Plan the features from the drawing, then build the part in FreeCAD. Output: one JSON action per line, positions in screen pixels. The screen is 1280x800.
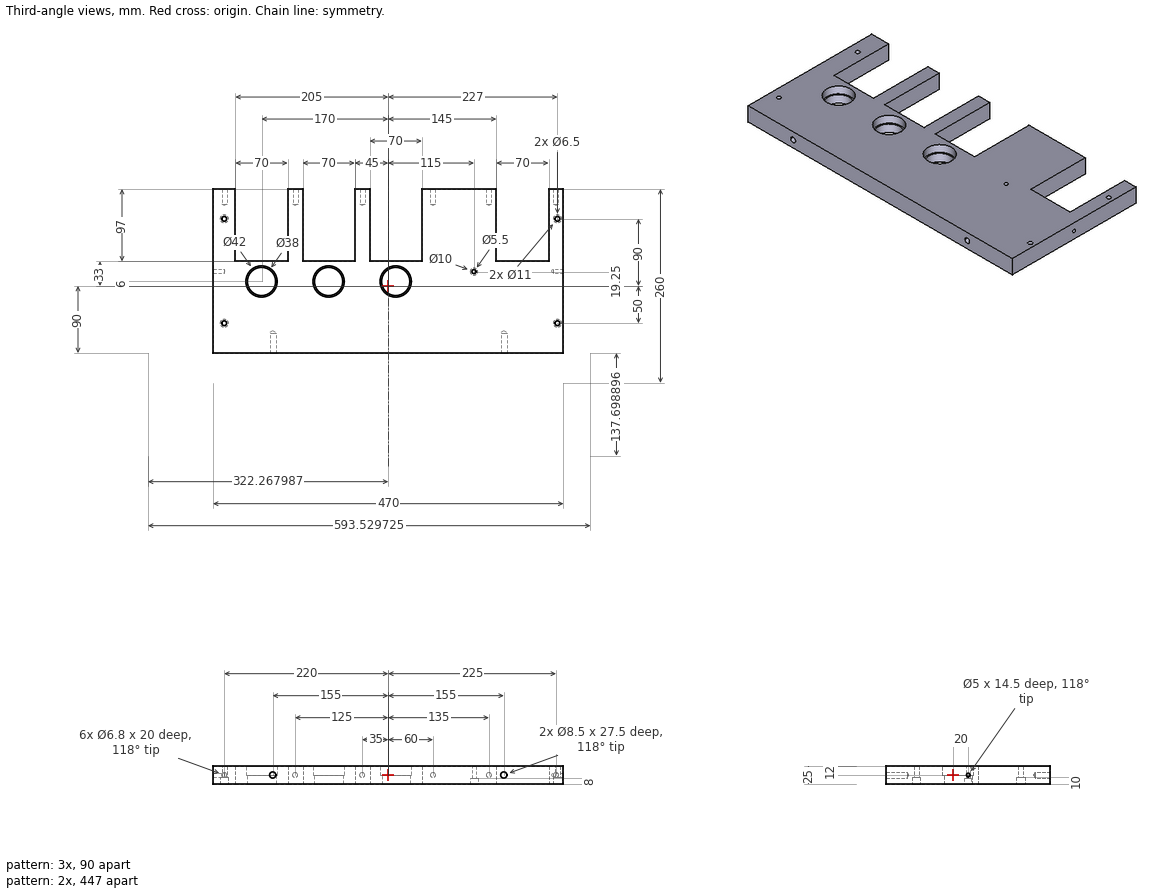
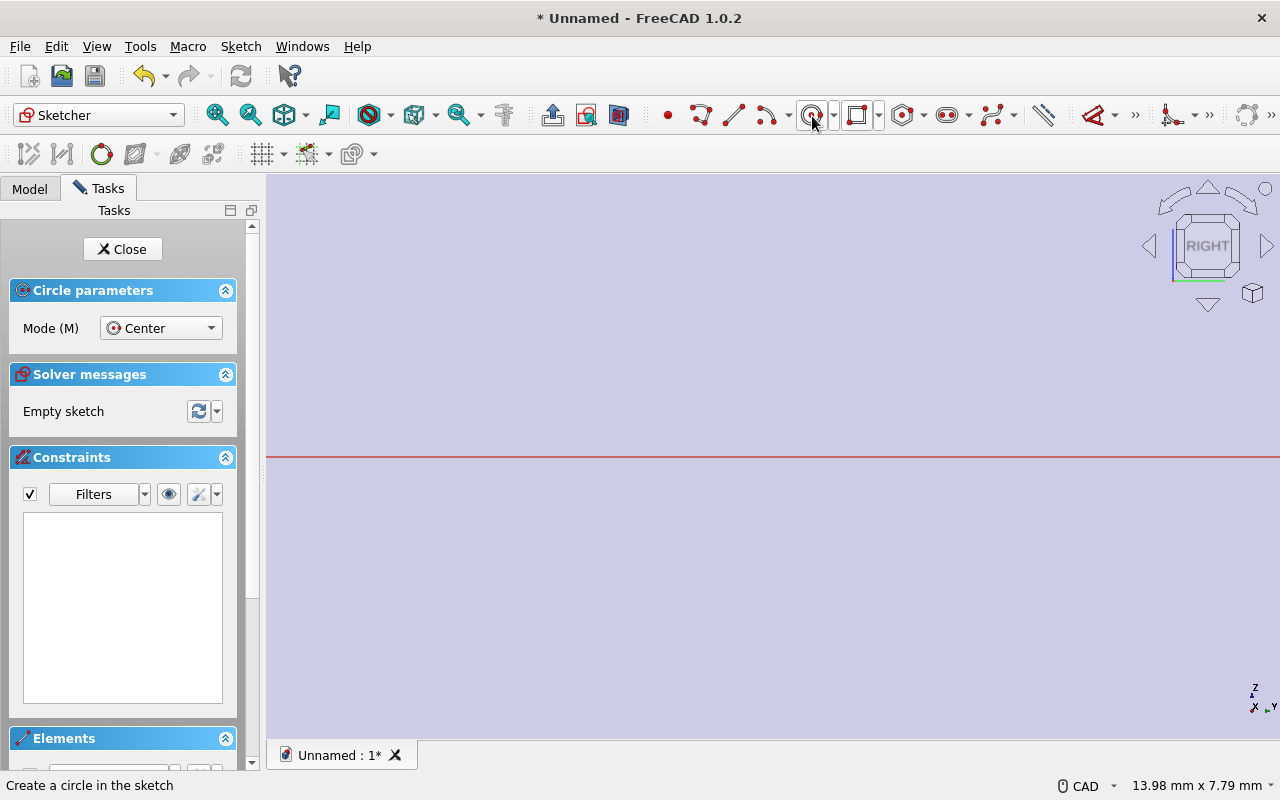
{"action": "left_click", "coordinate": [705, 456]}
{"action": "mouse_move", "coordinate": [833, 328]}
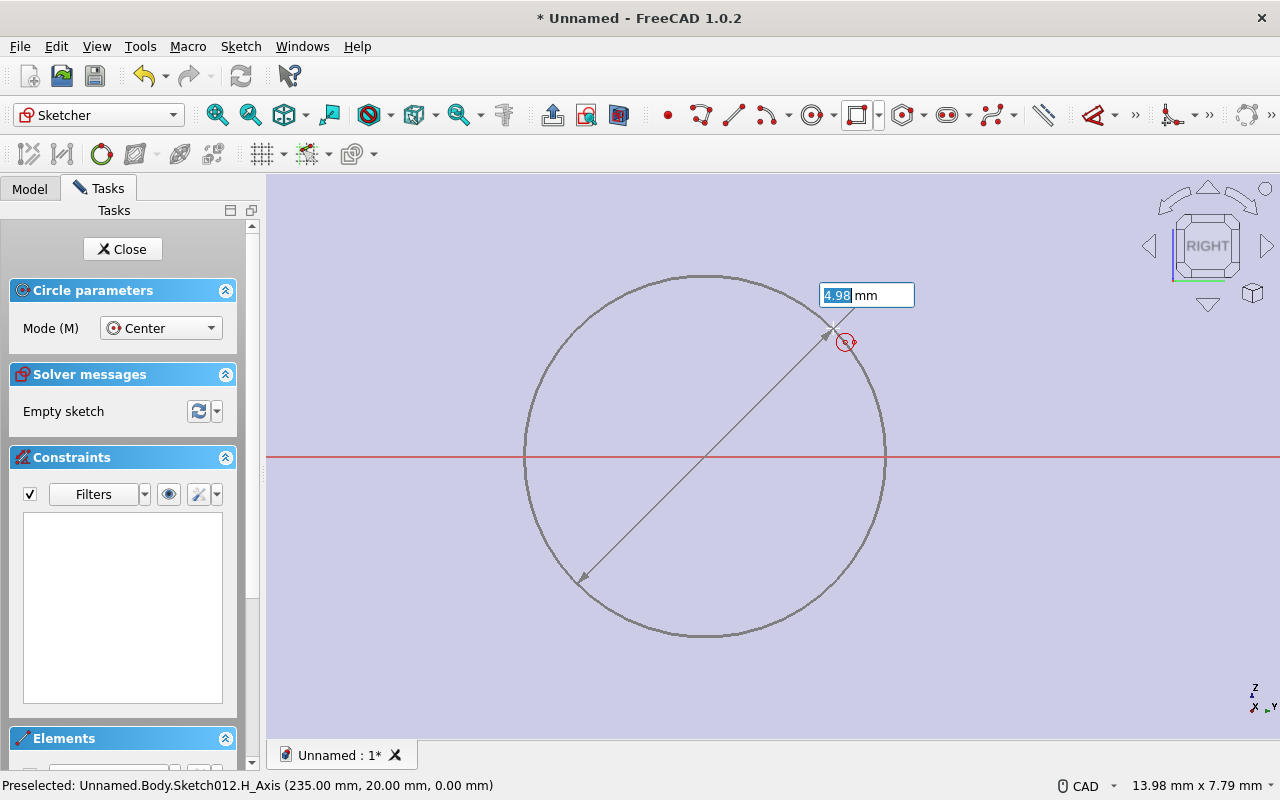
{"action": "type", "text": "5"}
{"action": "key", "text": "Return"}
{"action": "key", "text": "Escape"}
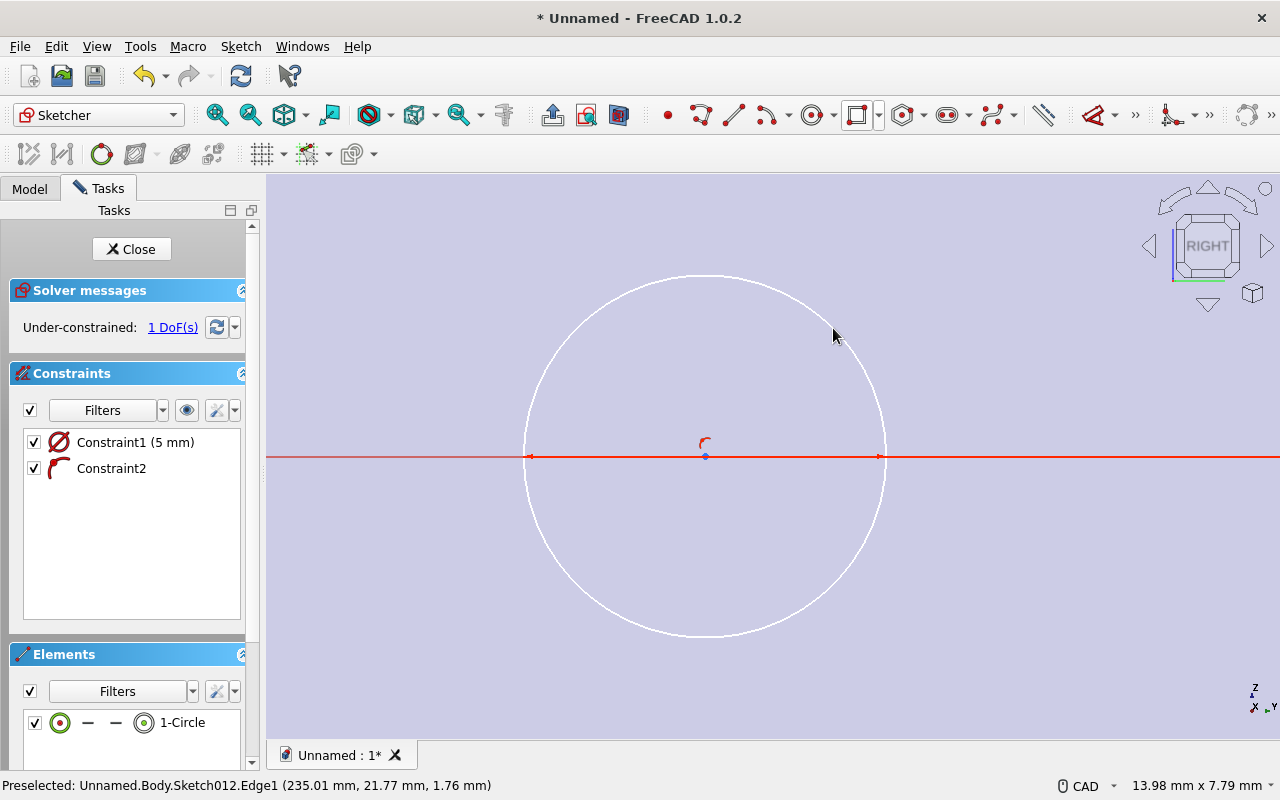
{"action": "left_click", "coordinate": [1092, 116]}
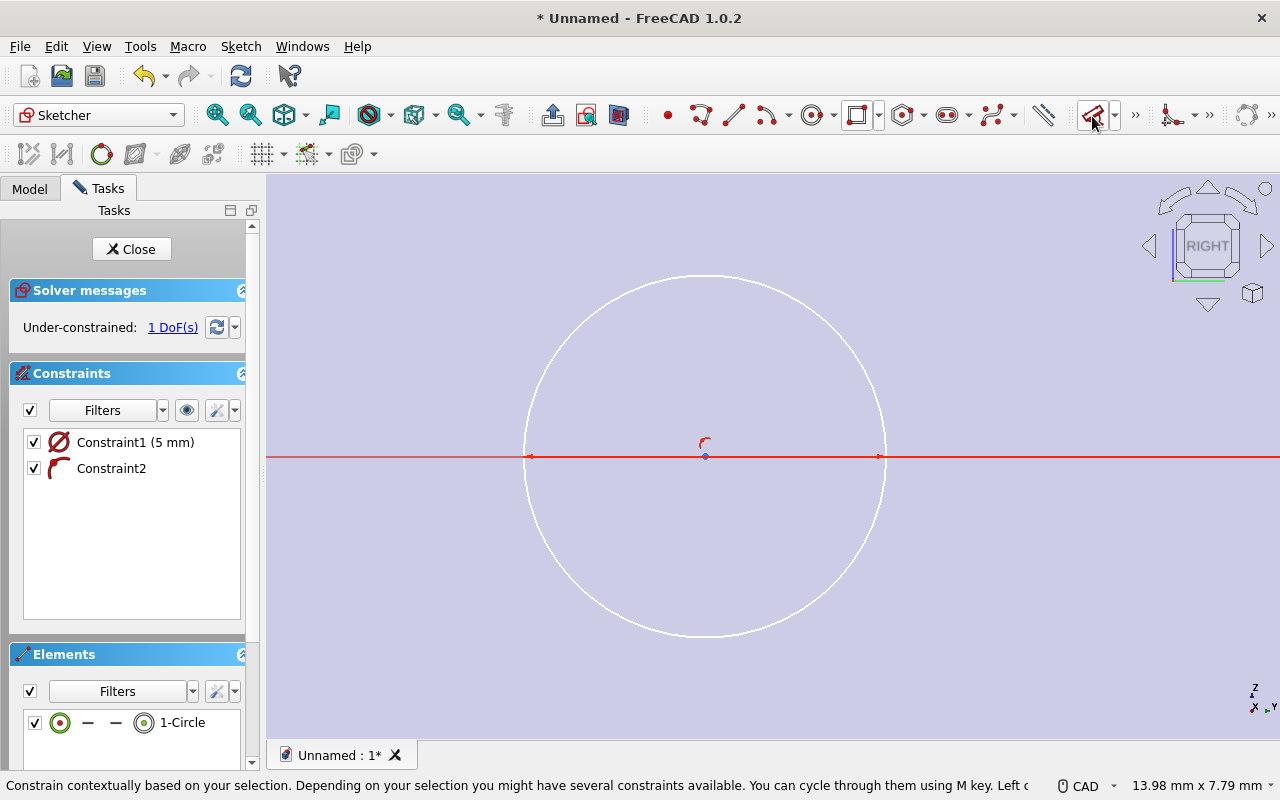
{"action": "left_click", "coordinate": [705, 456]}
{"action": "left_click", "coordinate": [499, 490]}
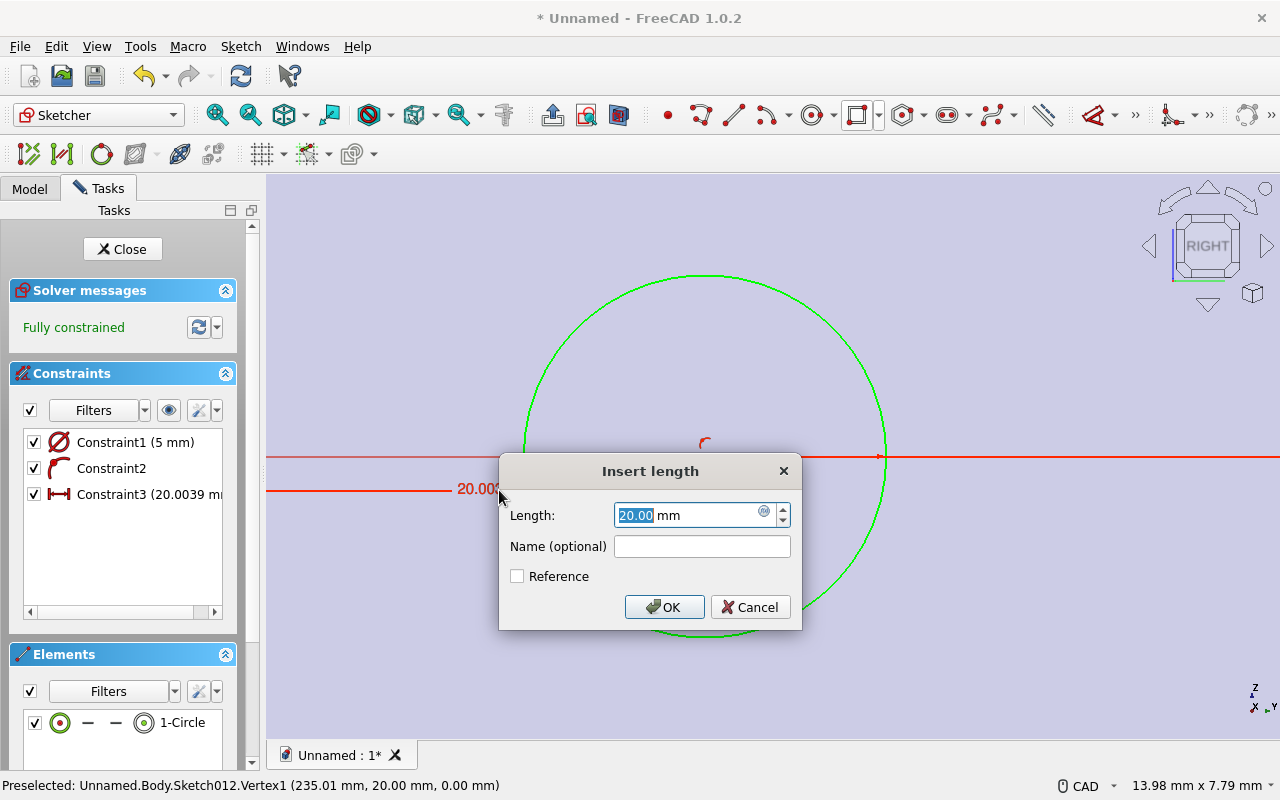
{"action": "type", "text": "20"}
{"action": "key", "text": "Return"}
{"action": "key", "text": "Escape"}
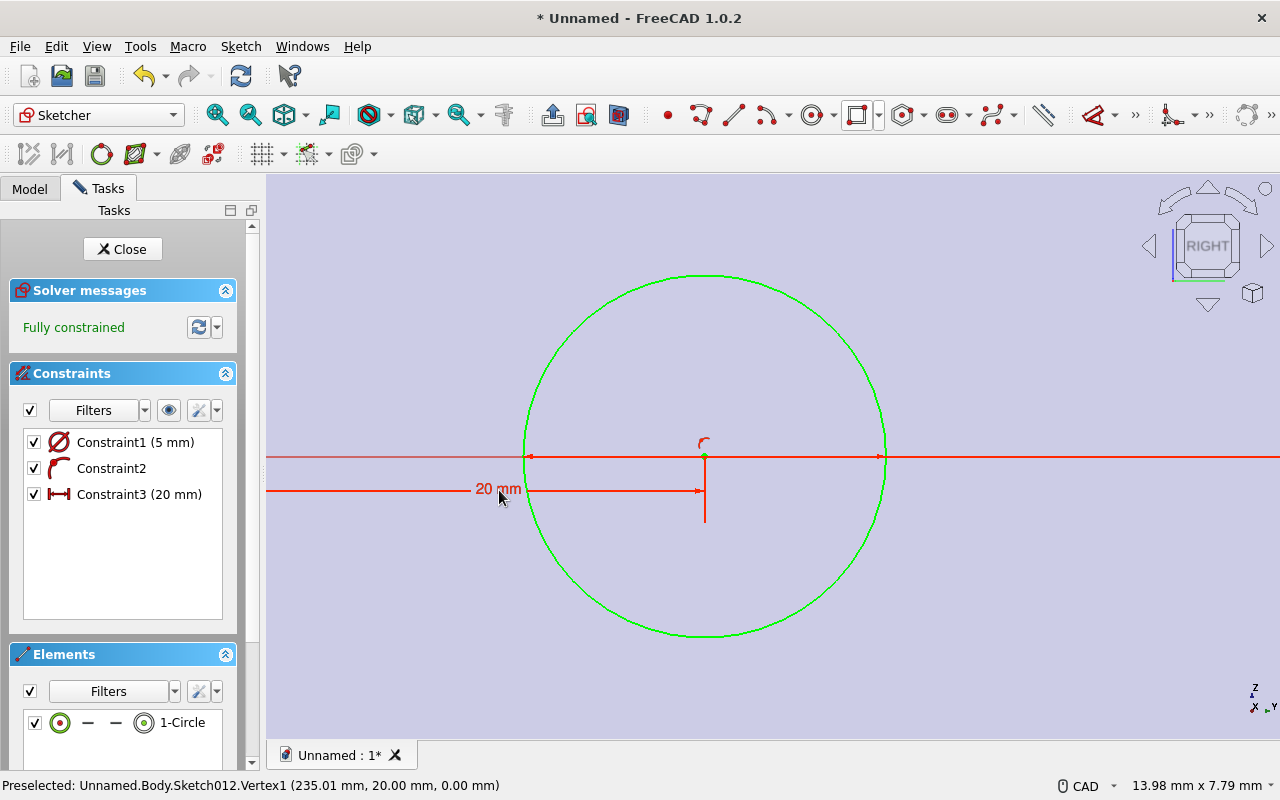
{"action": "left_click", "coordinate": [123, 249]}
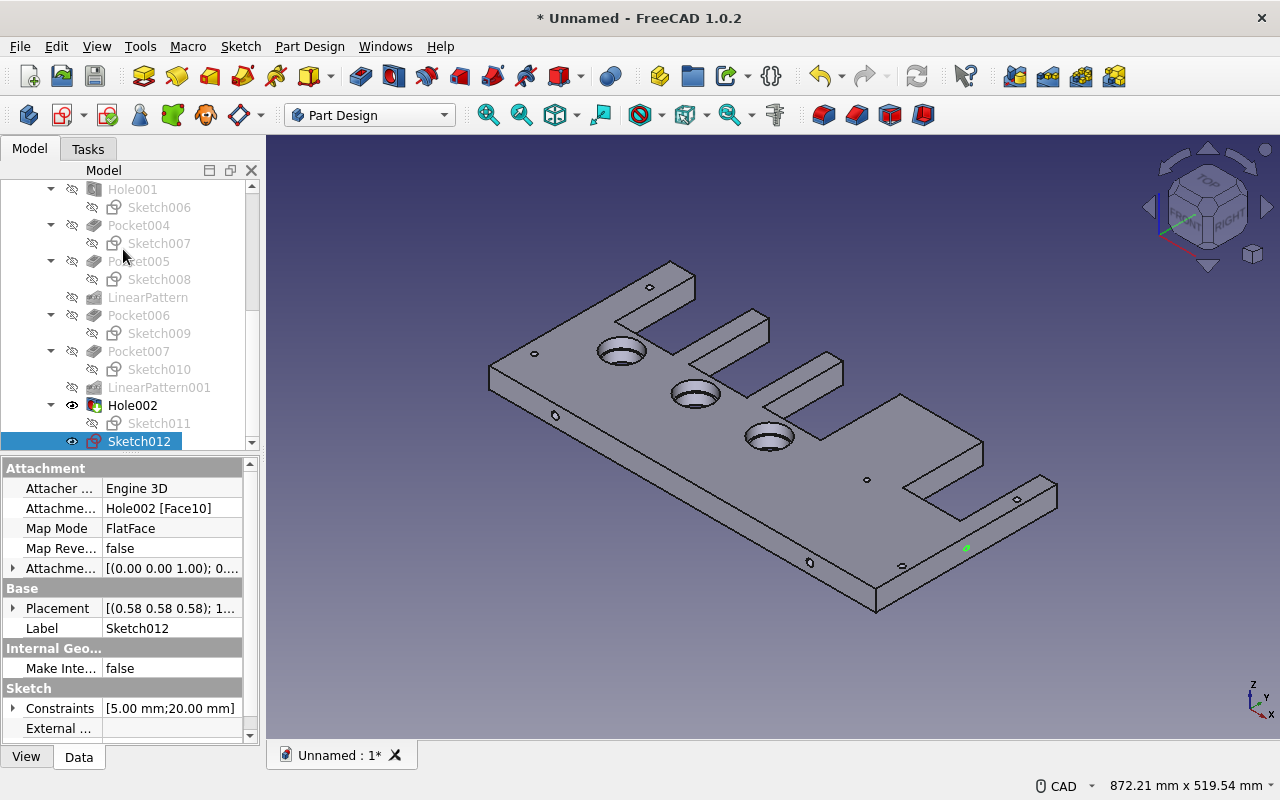
{"action": "left_click", "coordinate": [394, 76]}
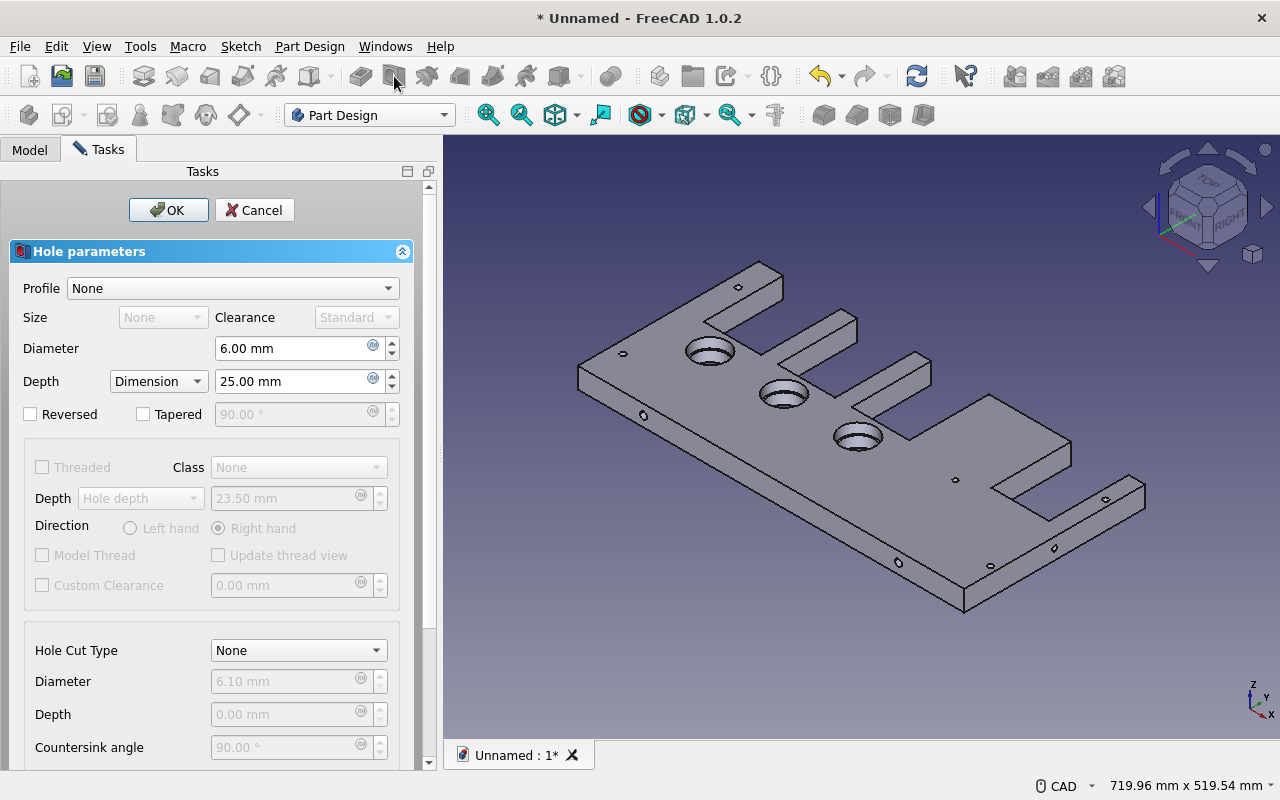
{"action": "triple_click", "coordinate": [300, 348]}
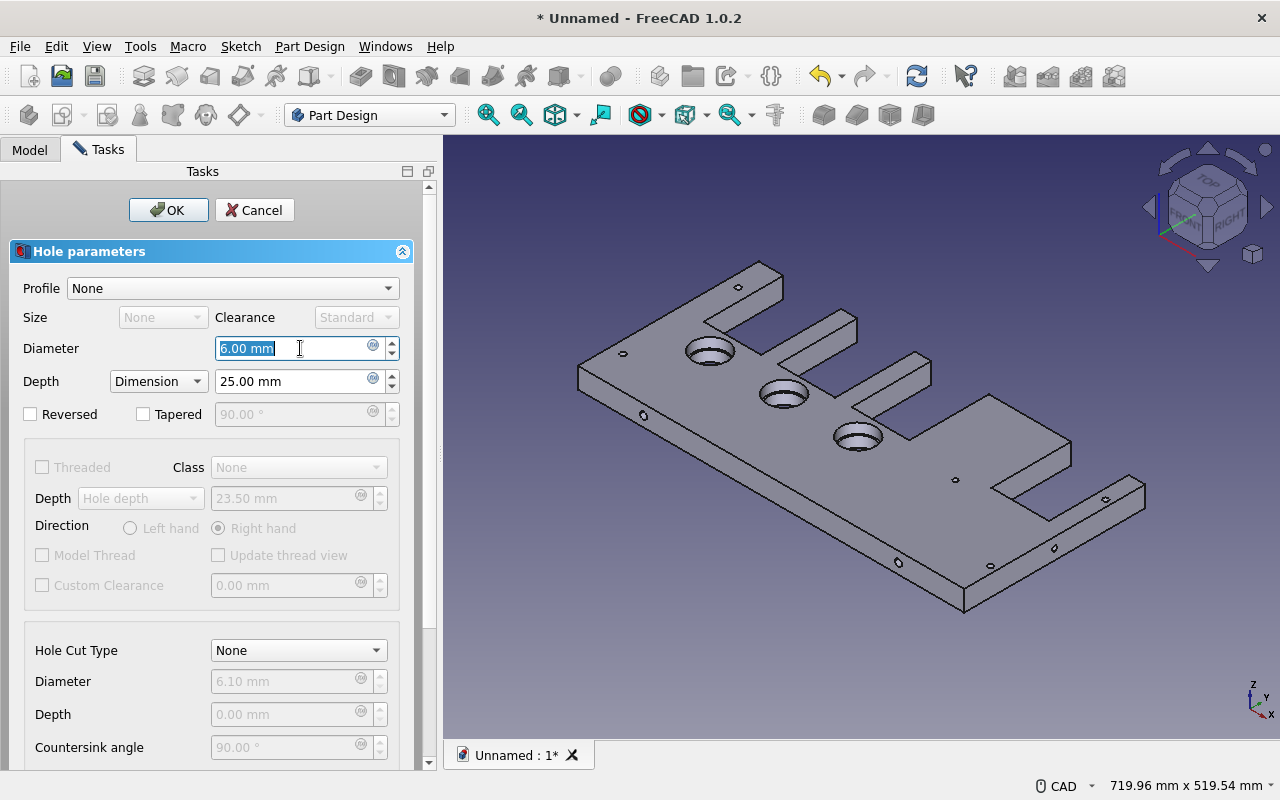
{"action": "type", "text": "5"}
{"action": "key", "text": "Tab"}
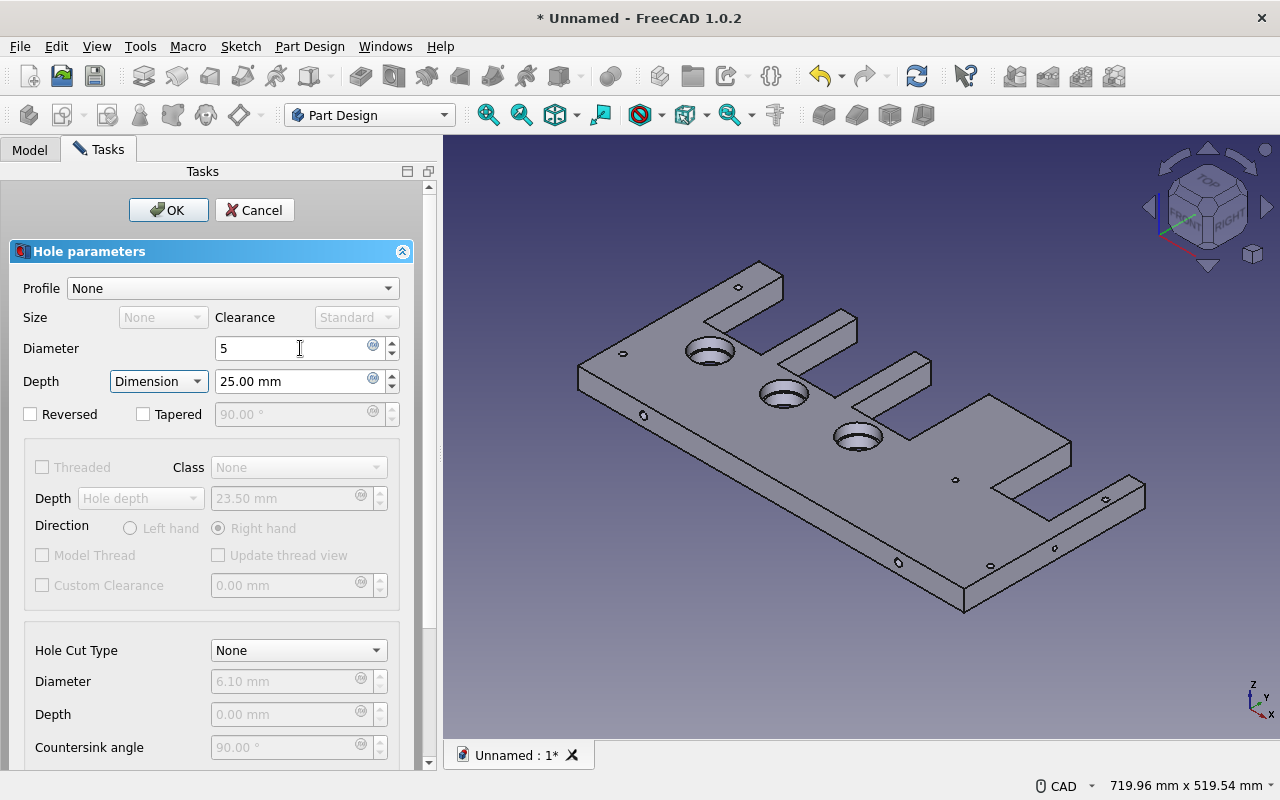
{"action": "triple_click", "coordinate": [300, 382]}